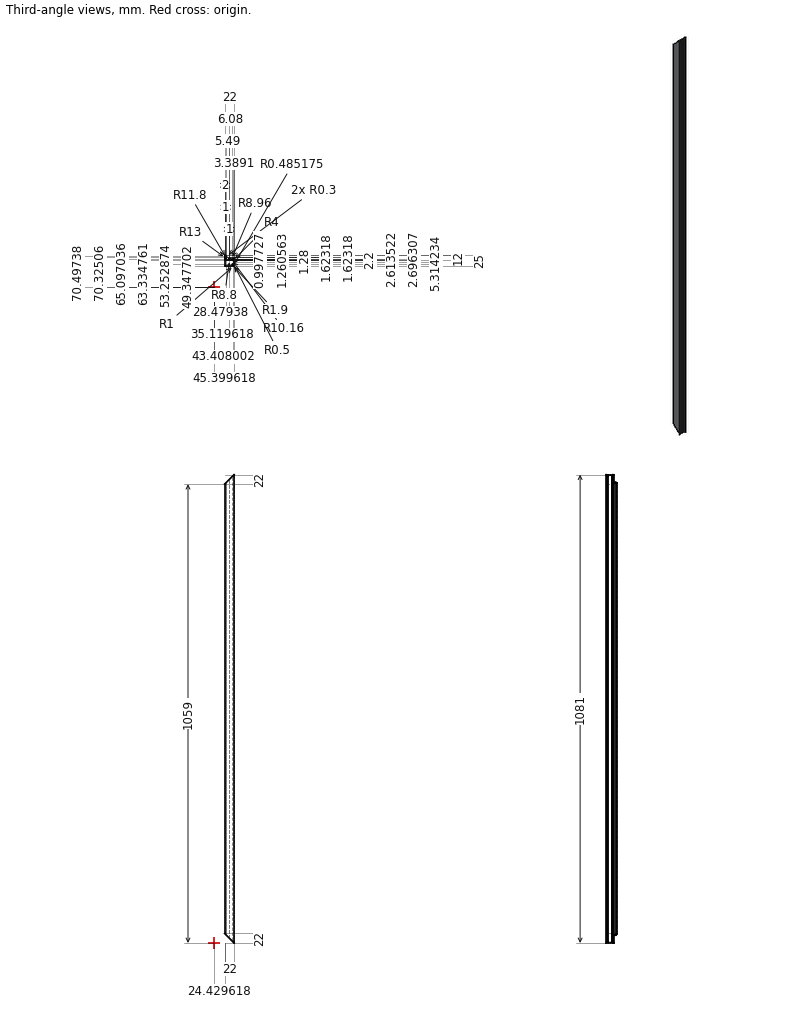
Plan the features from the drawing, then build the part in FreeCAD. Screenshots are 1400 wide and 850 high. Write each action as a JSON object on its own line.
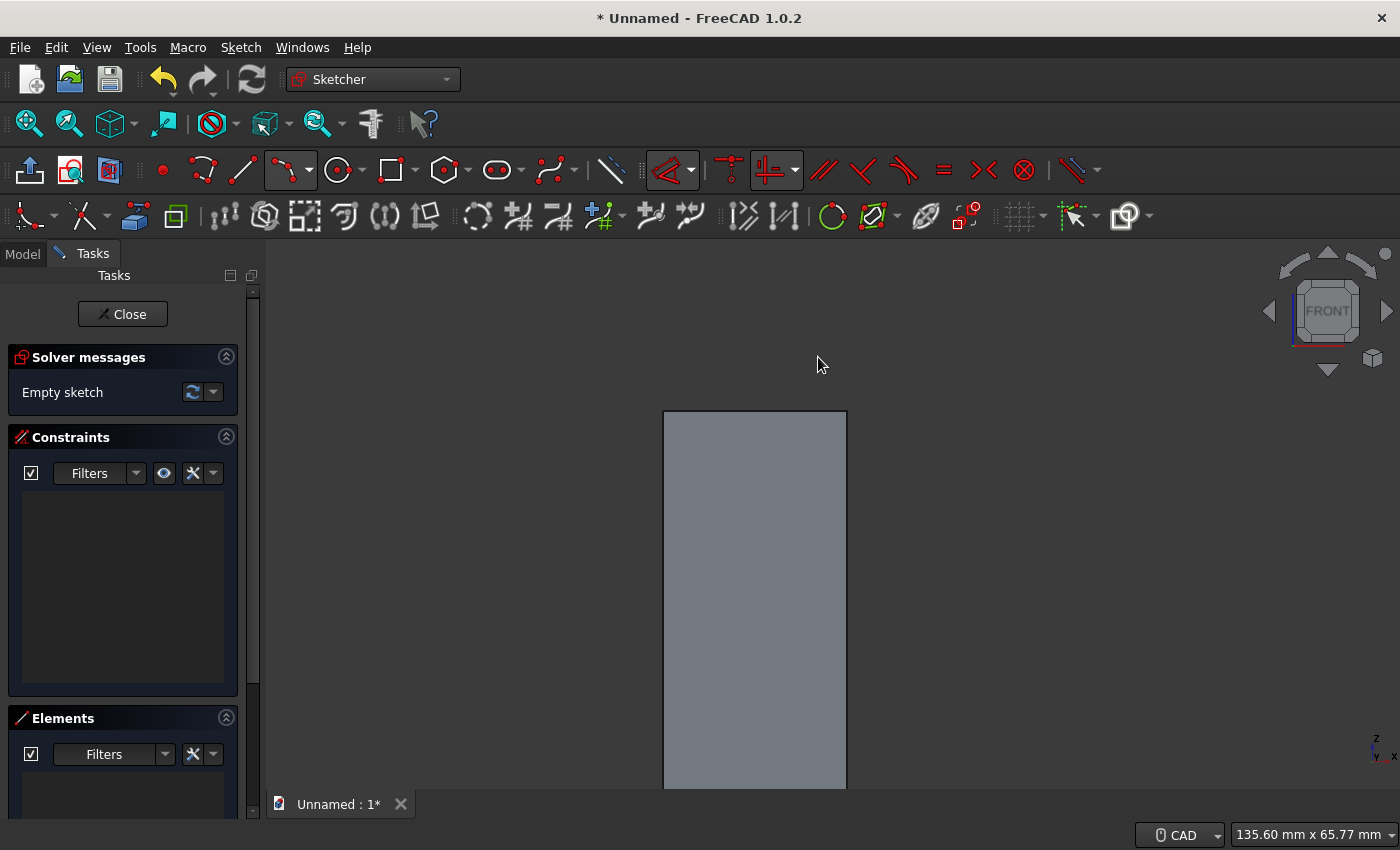
{"action": "scroll", "coordinate": [745, 489], "scroll_direction": "up", "scroll_amount": 3}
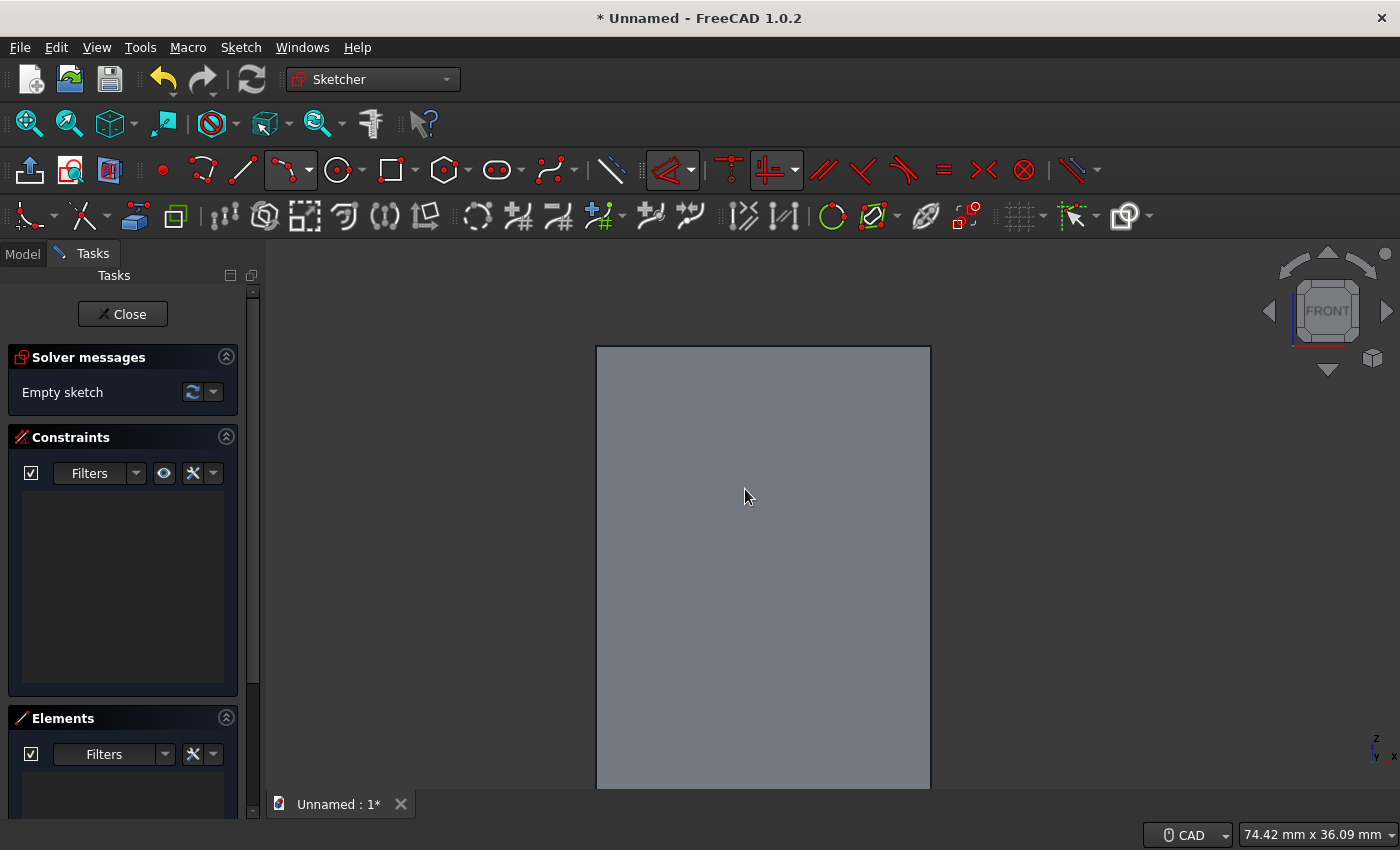
{"action": "left_click", "coordinate": [204, 170]}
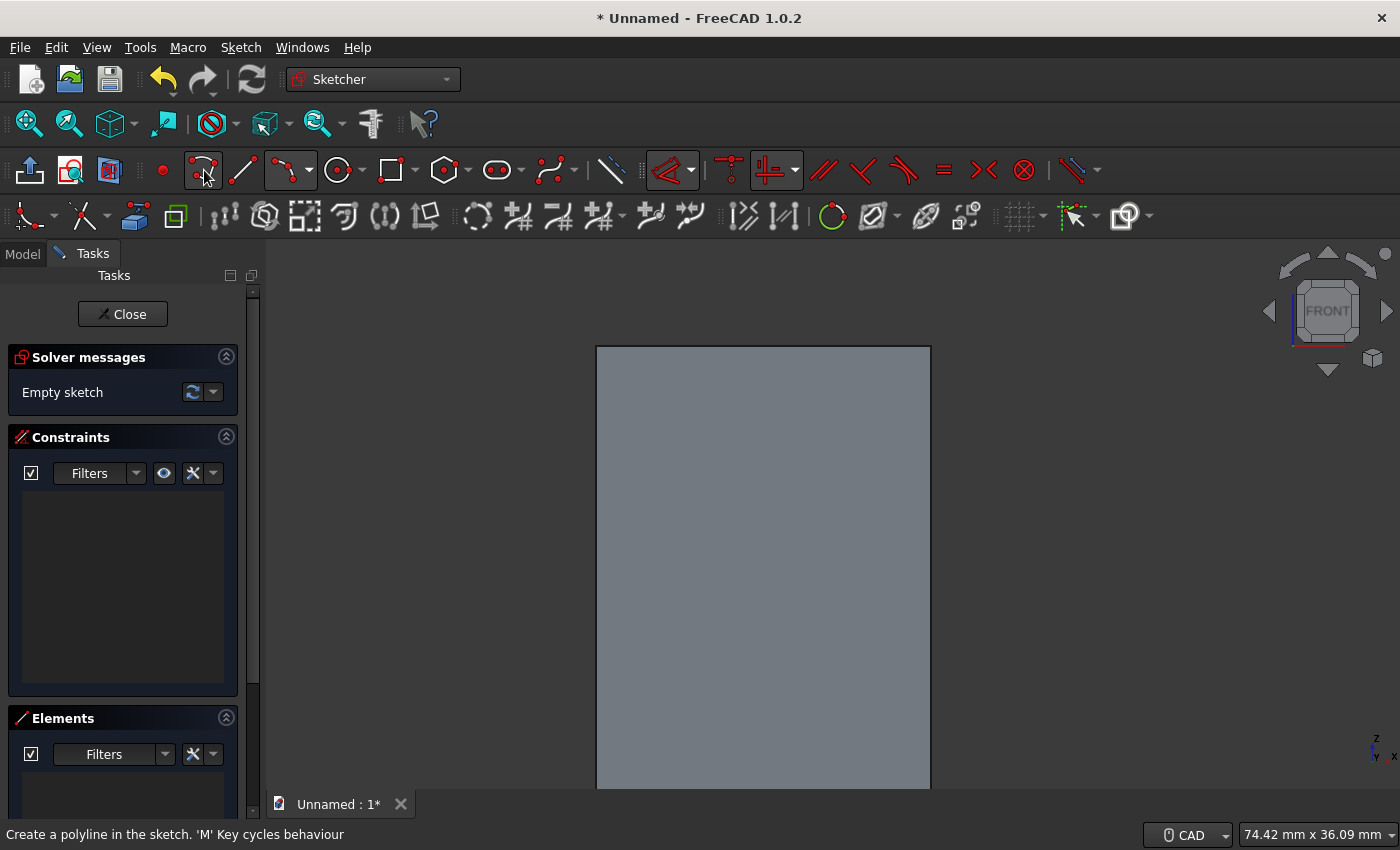
{"action": "left_click", "coordinate": [596, 681]}
{"action": "left_click", "coordinate": [931, 346]}
{"action": "left_click", "coordinate": [596, 346]}
{"action": "left_click", "coordinate": [596, 682]}
{"action": "key", "text": "Escape"}
{"action": "key", "text": "Escape"}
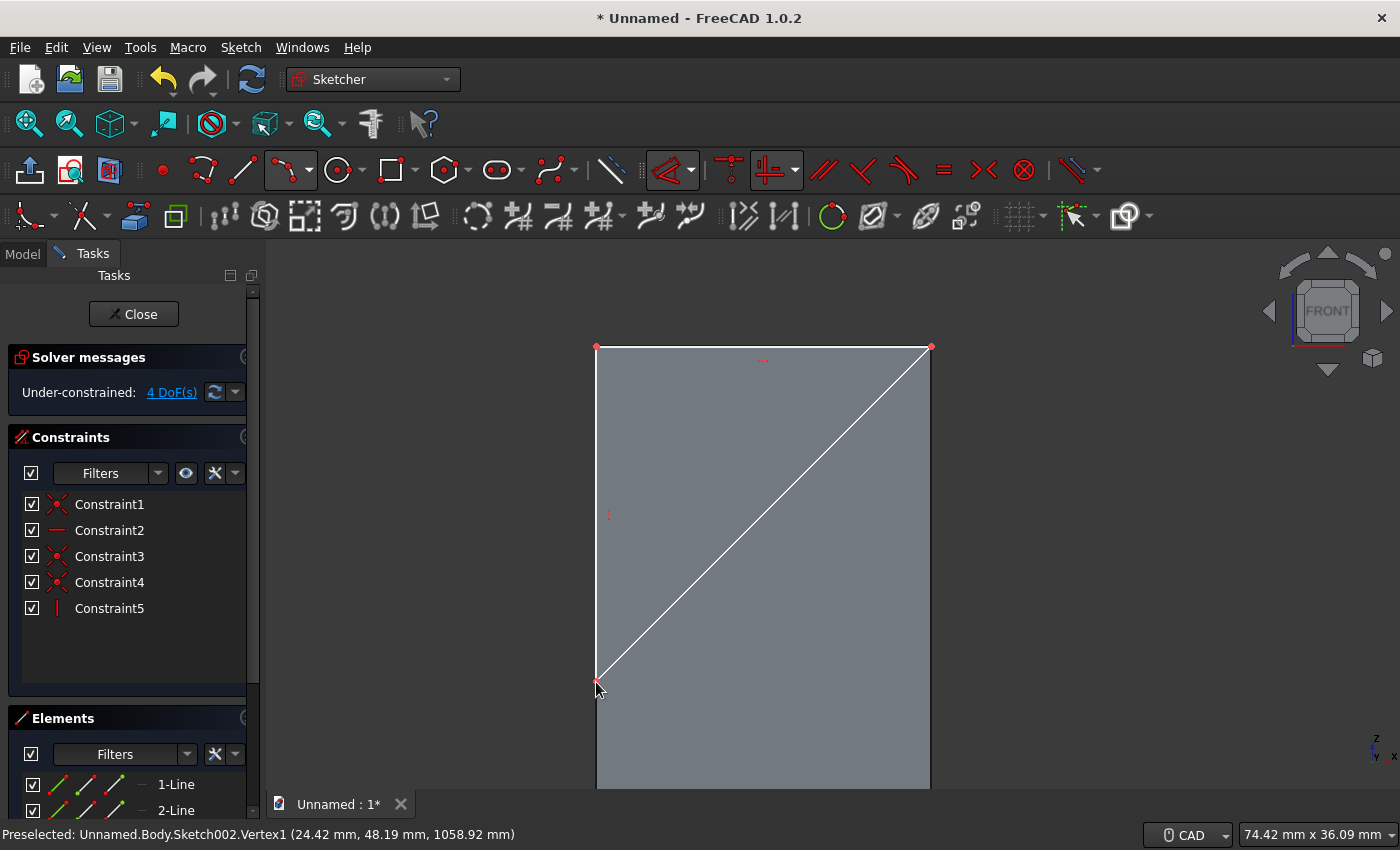
{"action": "left_click", "coordinate": [830, 347]}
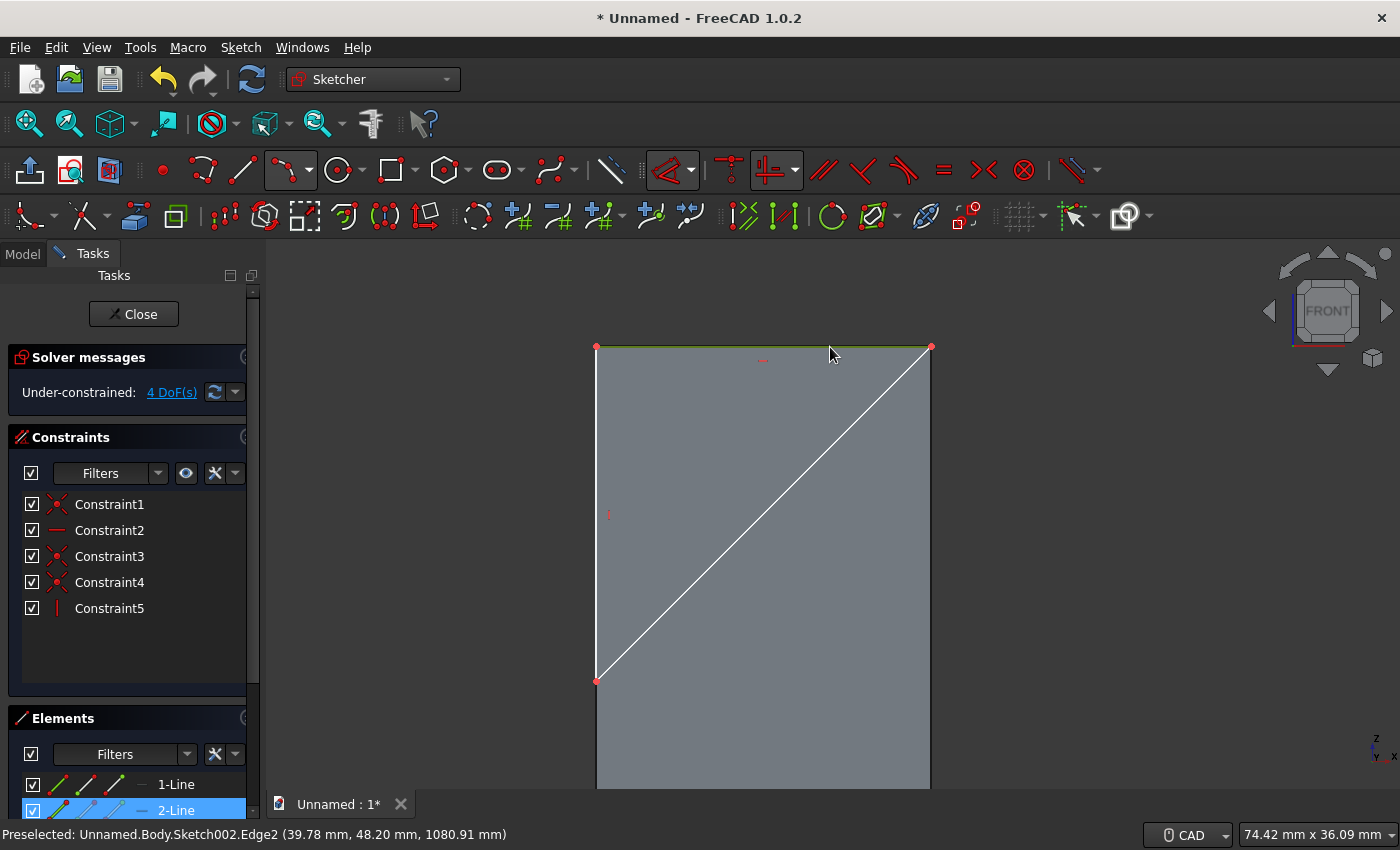
{"action": "left_click", "coordinate": [694, 170]}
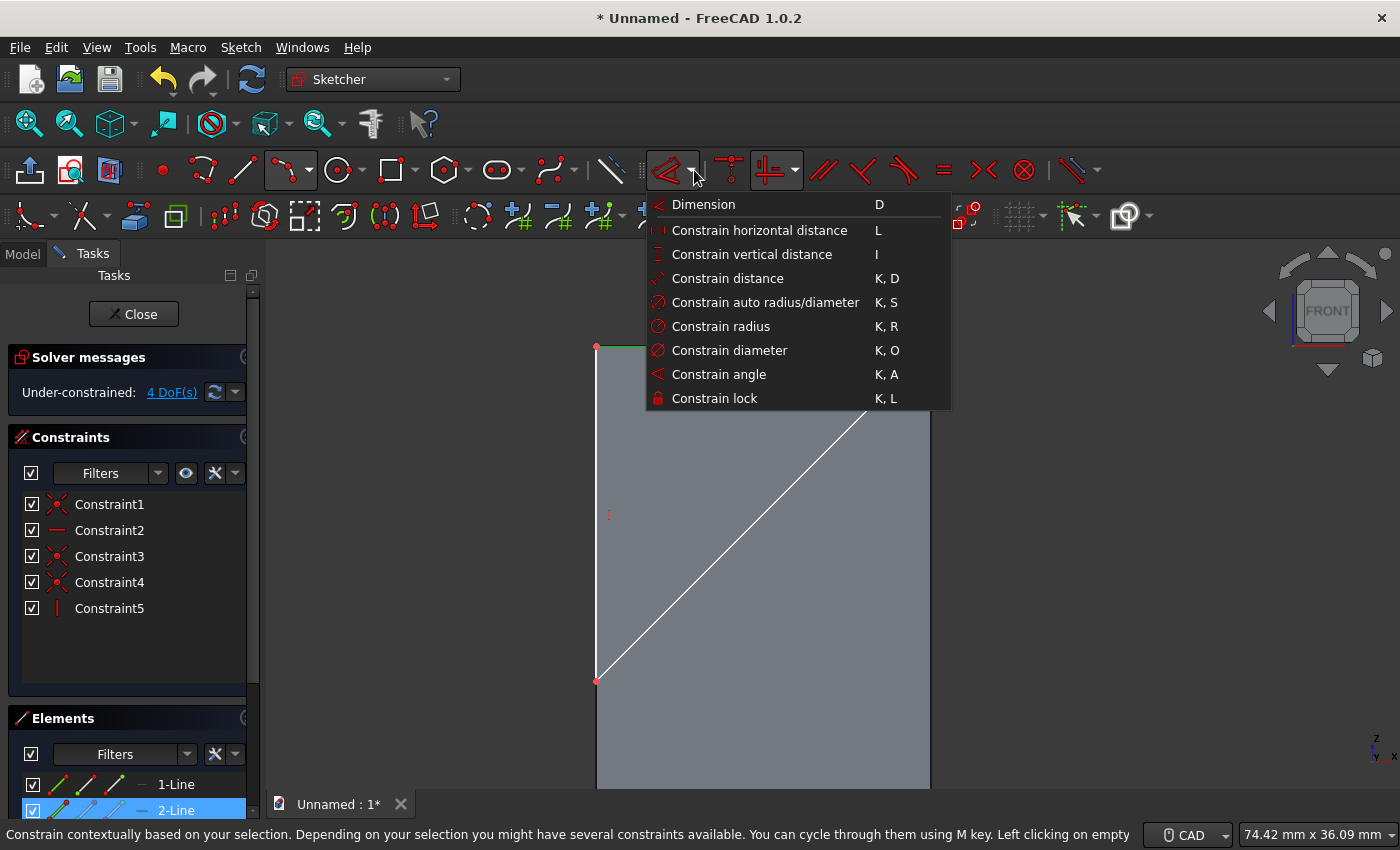
{"action": "left_click", "coordinate": [799, 230]}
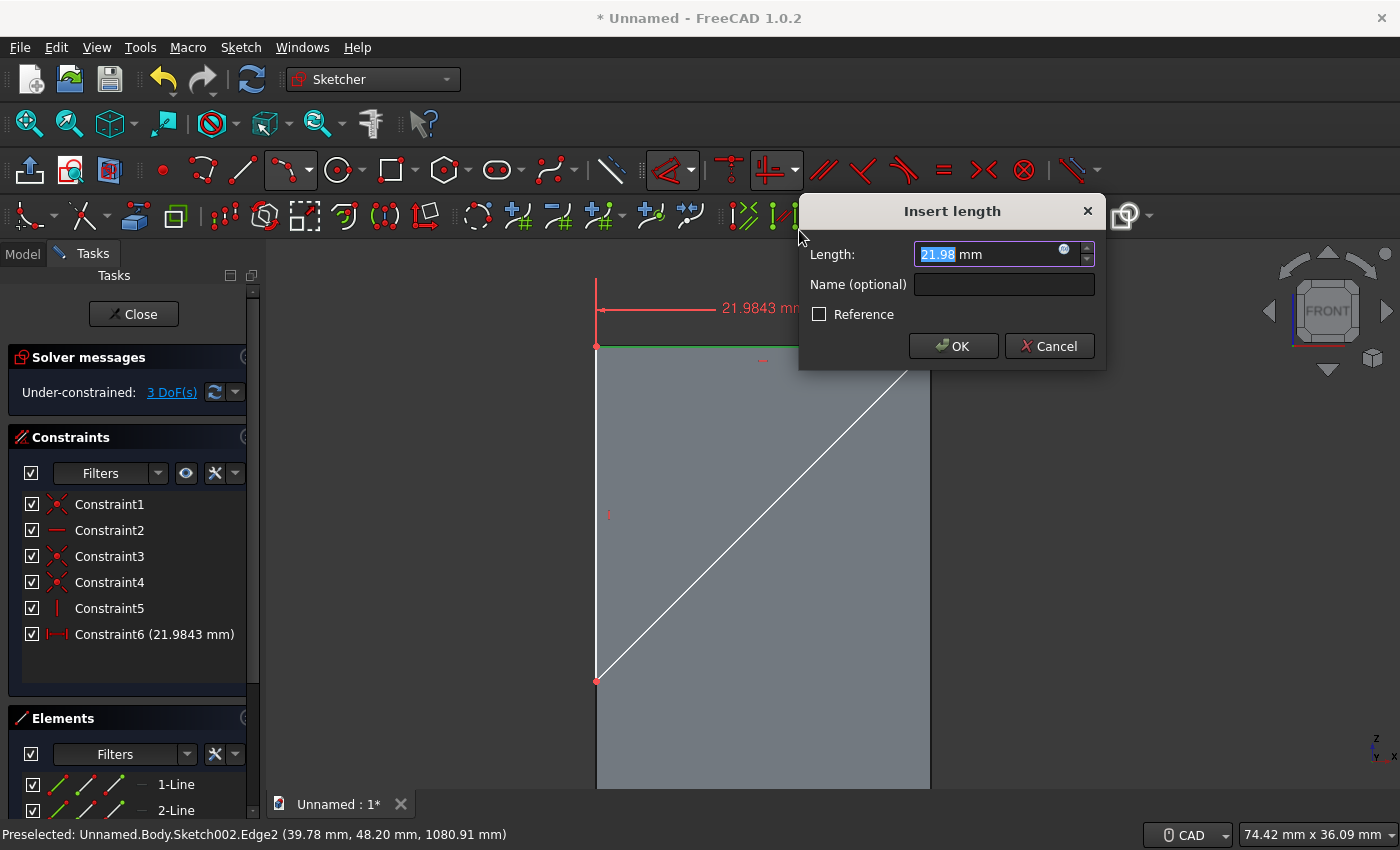
{"action": "type", "text": "22"}
{"action": "key", "text": "Return"}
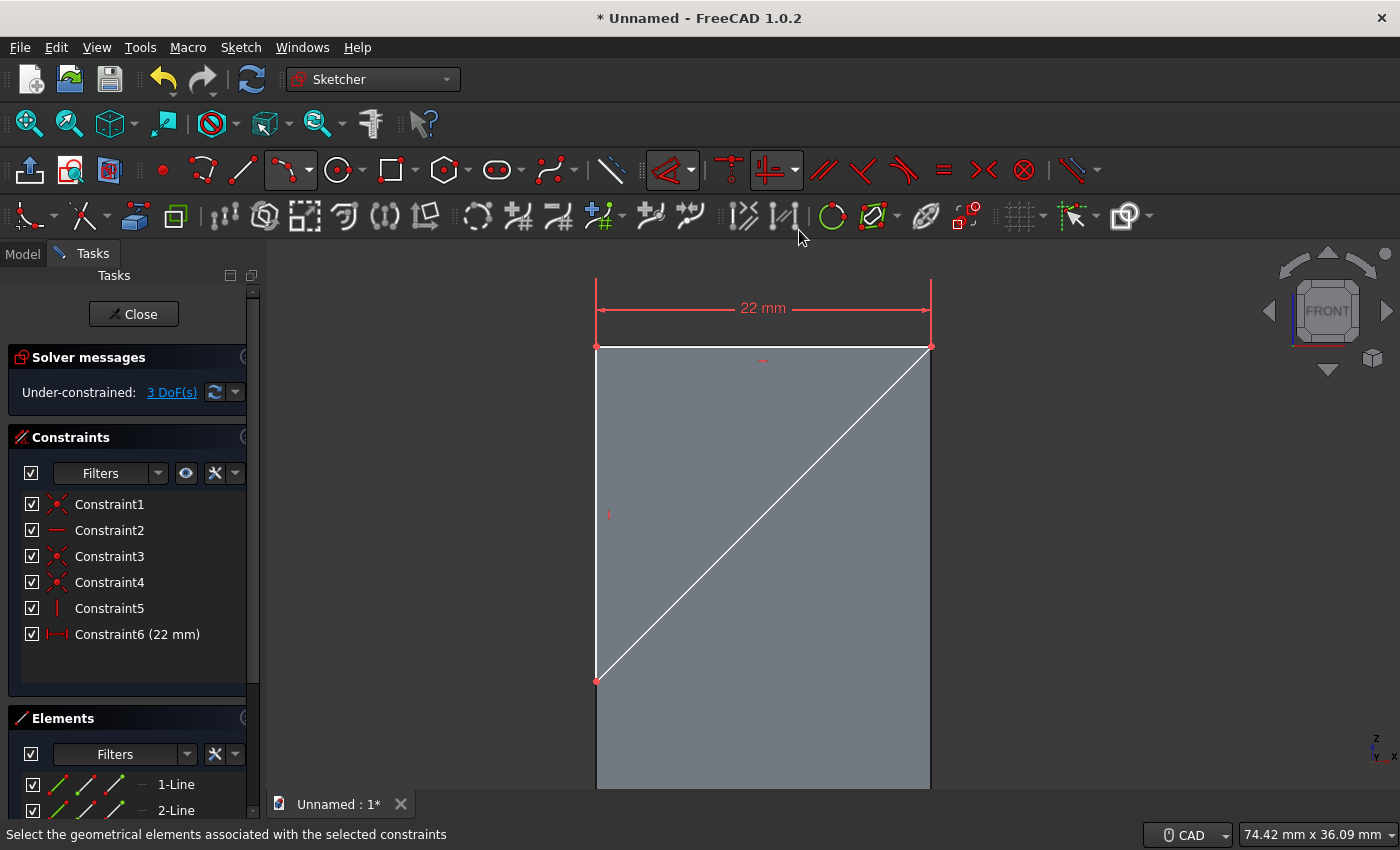
{"action": "left_click", "coordinate": [596, 448]}